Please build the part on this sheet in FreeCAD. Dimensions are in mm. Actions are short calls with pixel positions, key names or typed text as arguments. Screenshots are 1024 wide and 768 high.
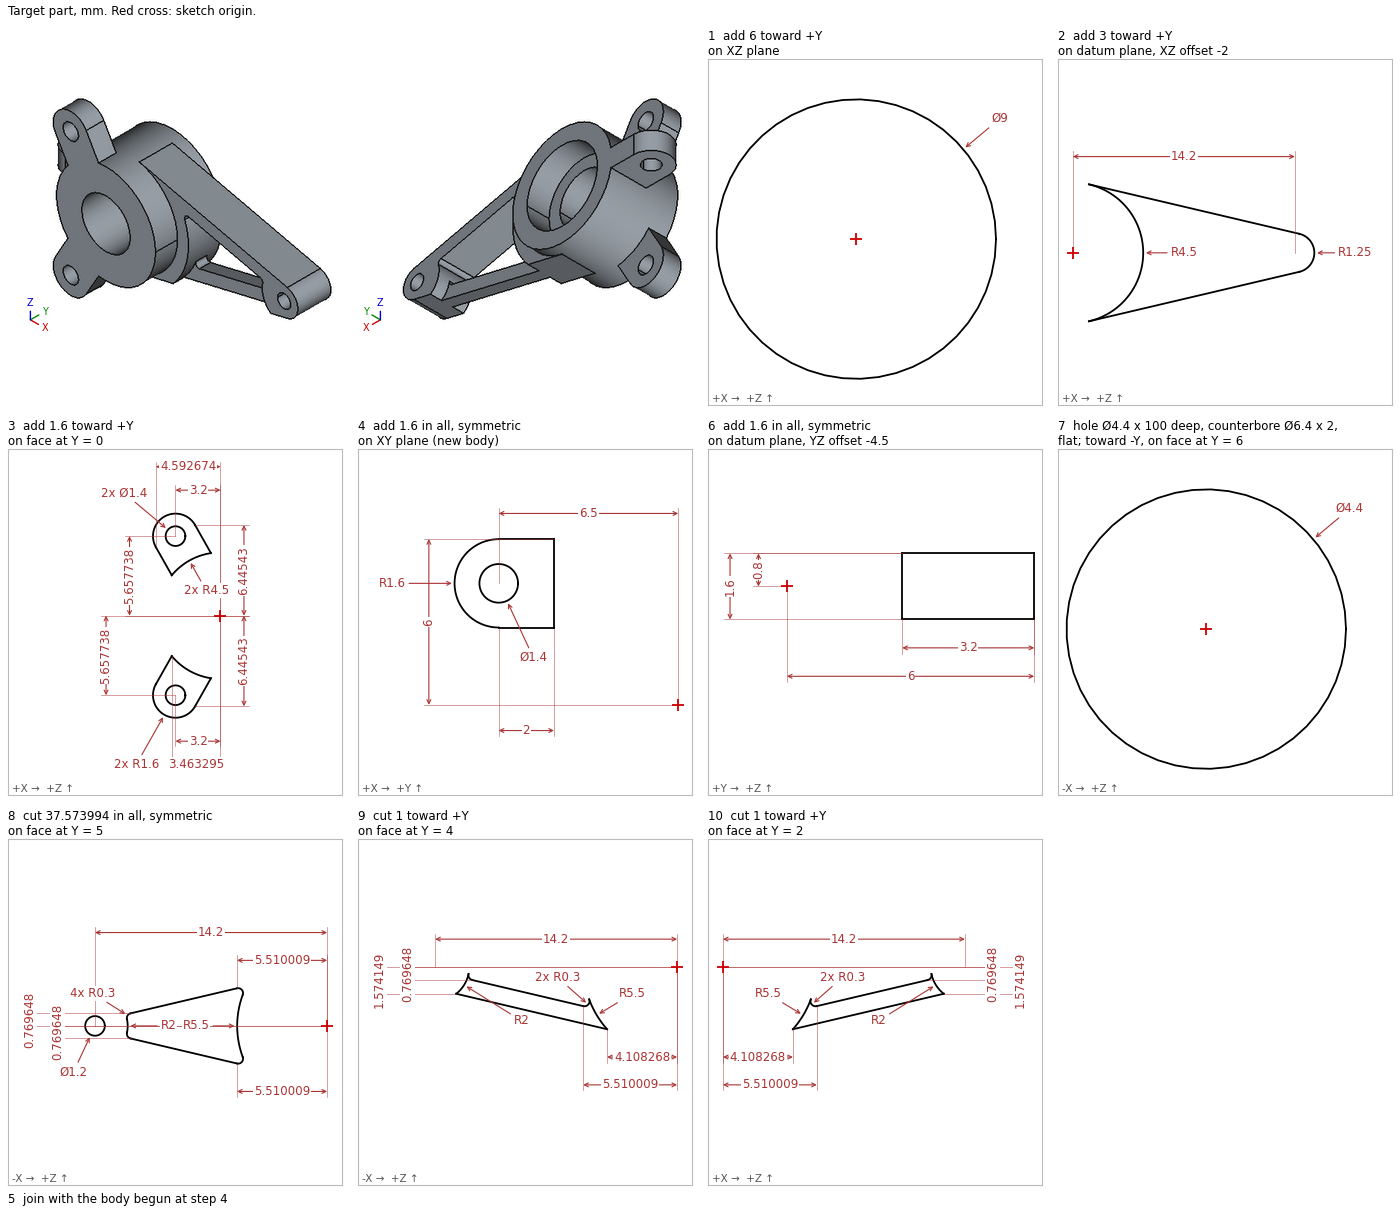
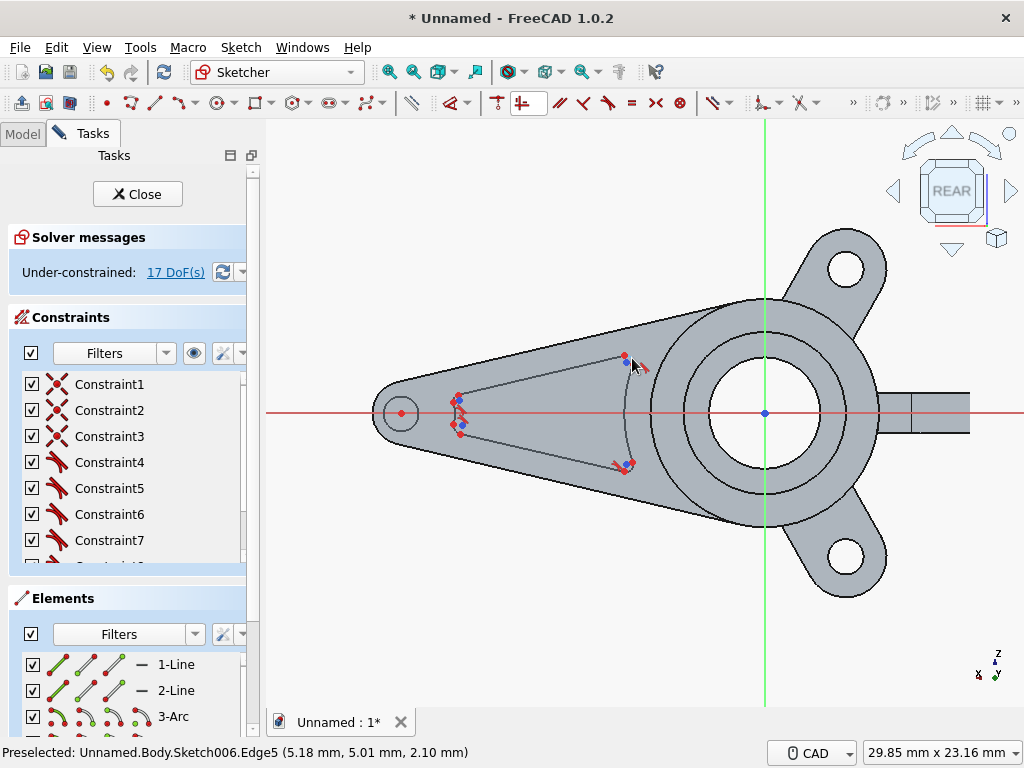
scroll(454, 398, up, 6)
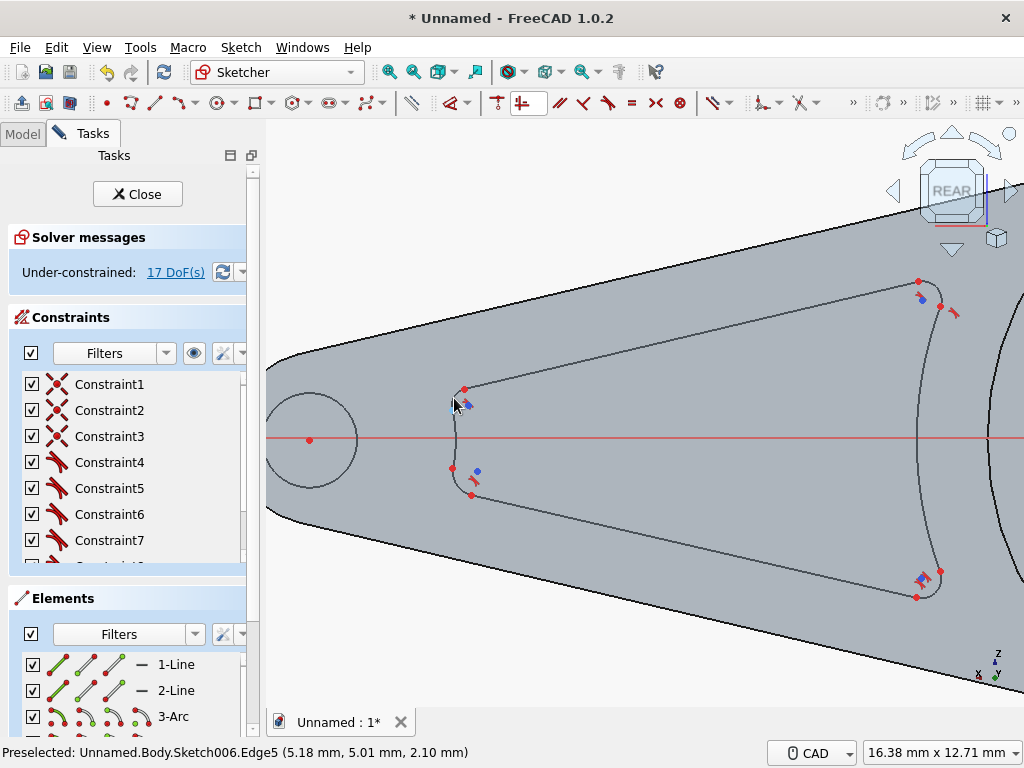
click(454, 397)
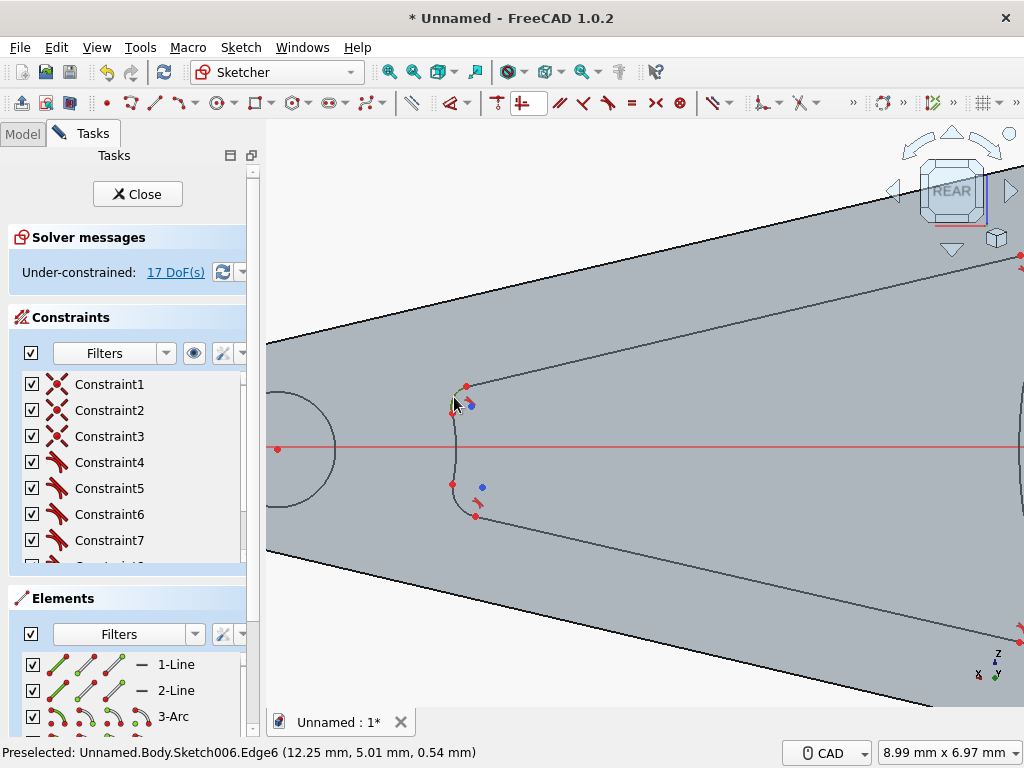
click(456, 463)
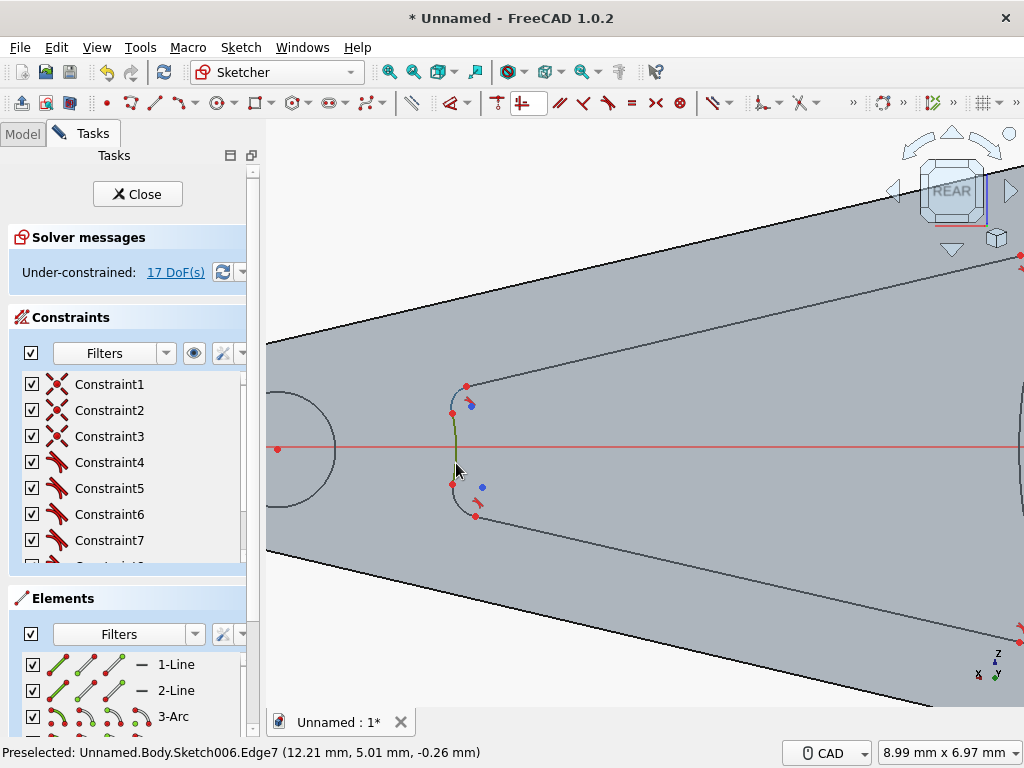
key(t)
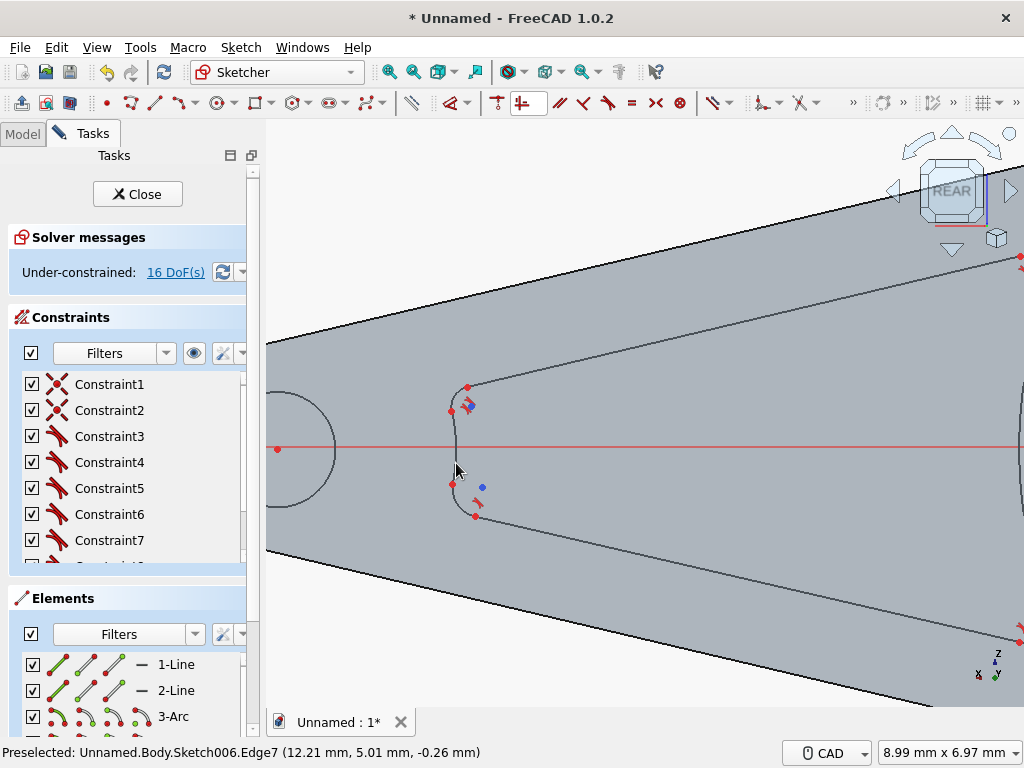
click(456, 462)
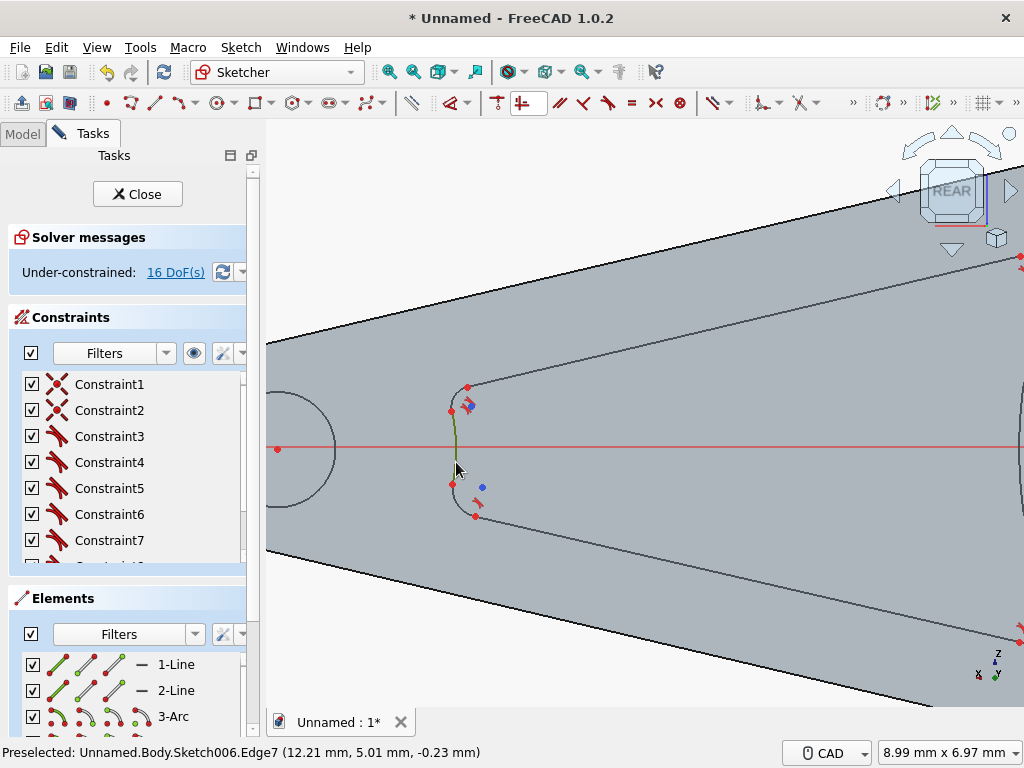
click(454, 497)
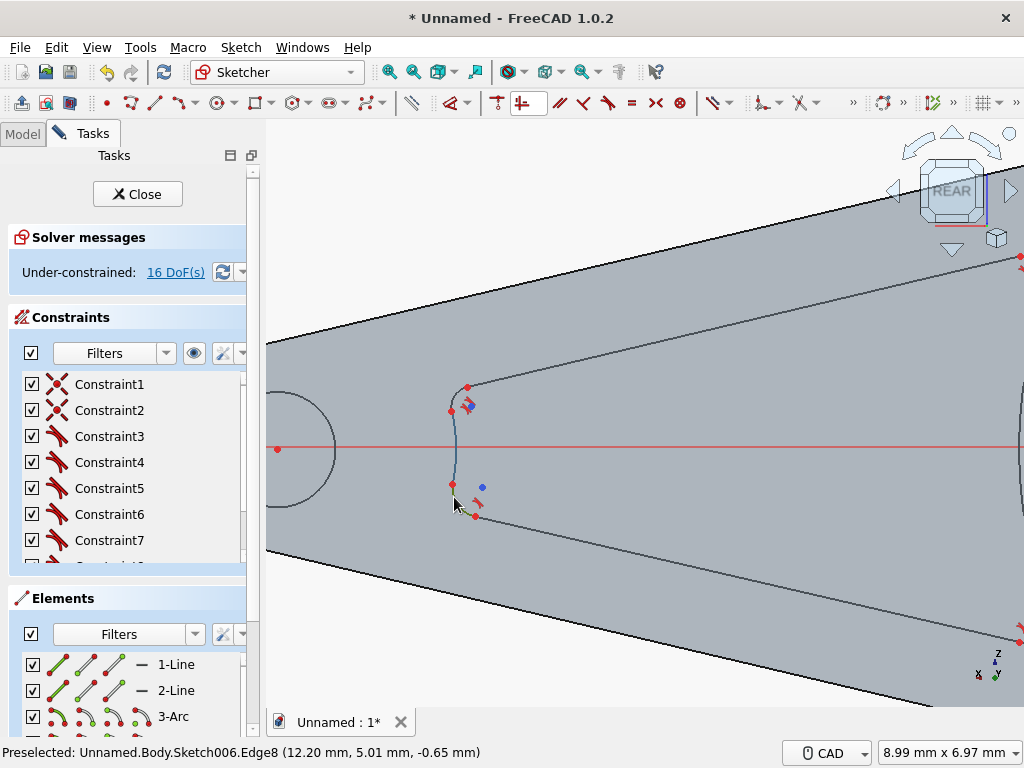
click(608, 104)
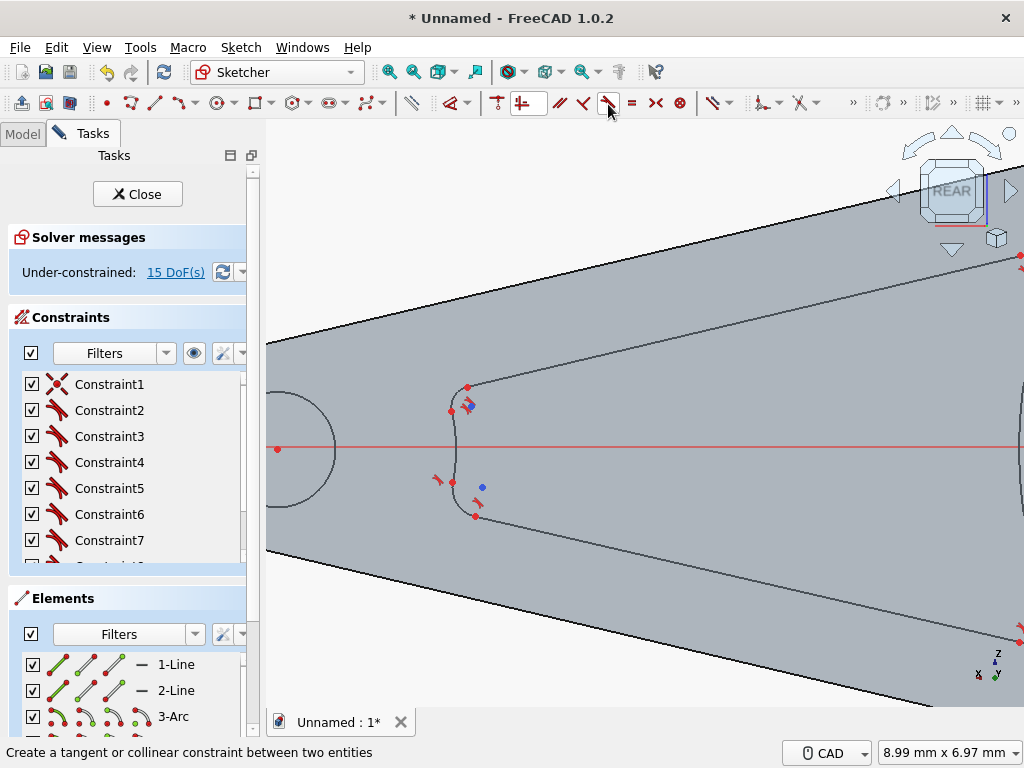
scroll(454, 398, down, 6)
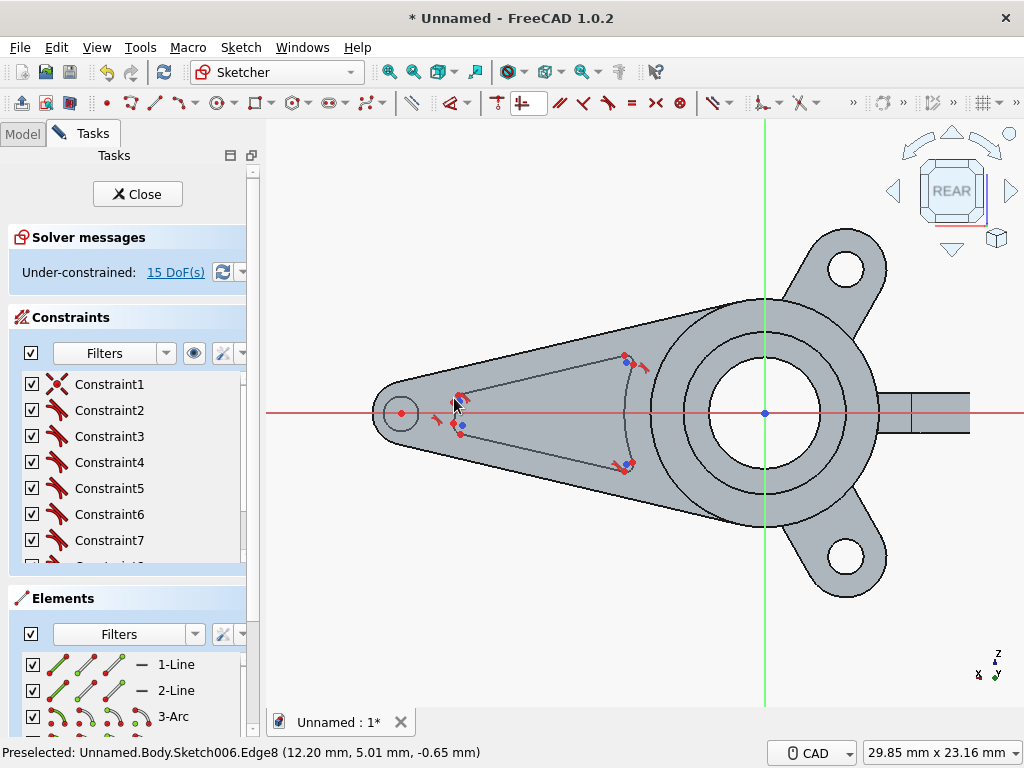
scroll(765, 413, up, 10)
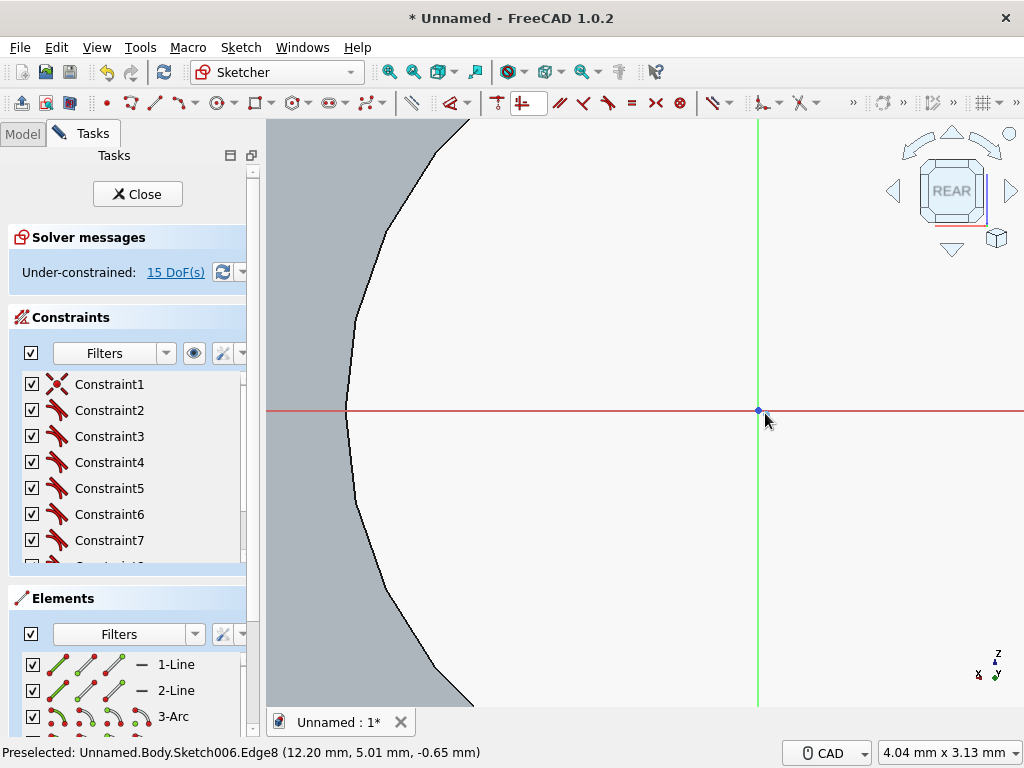
drag(748, 401, 777, 425)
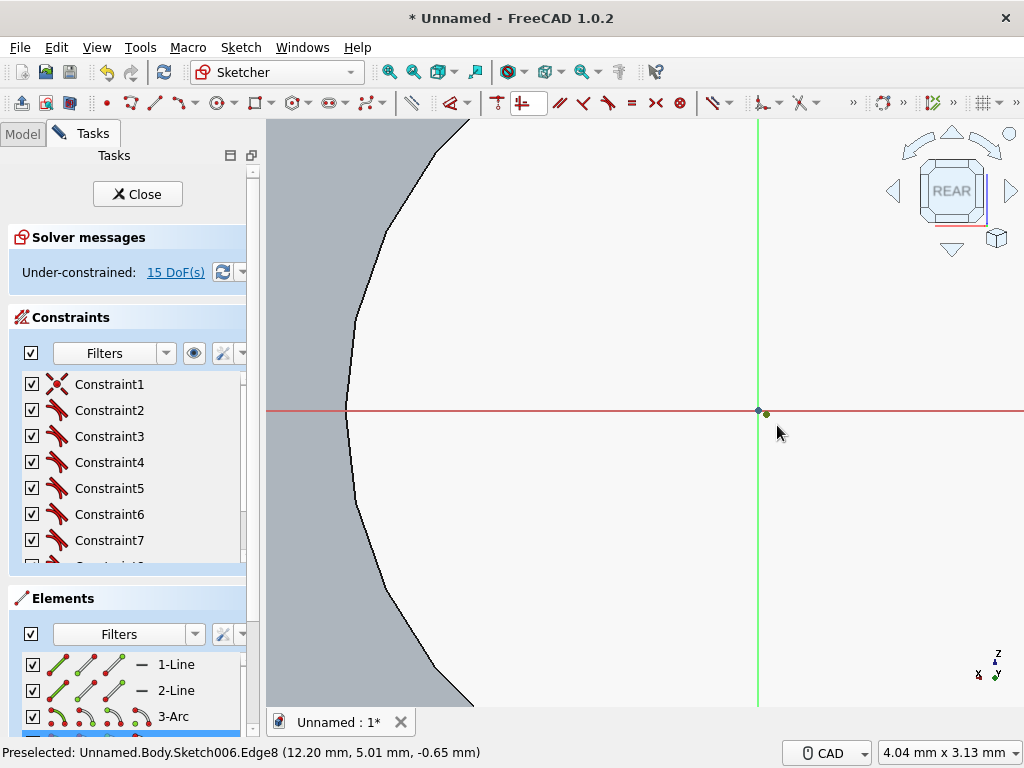
key(c)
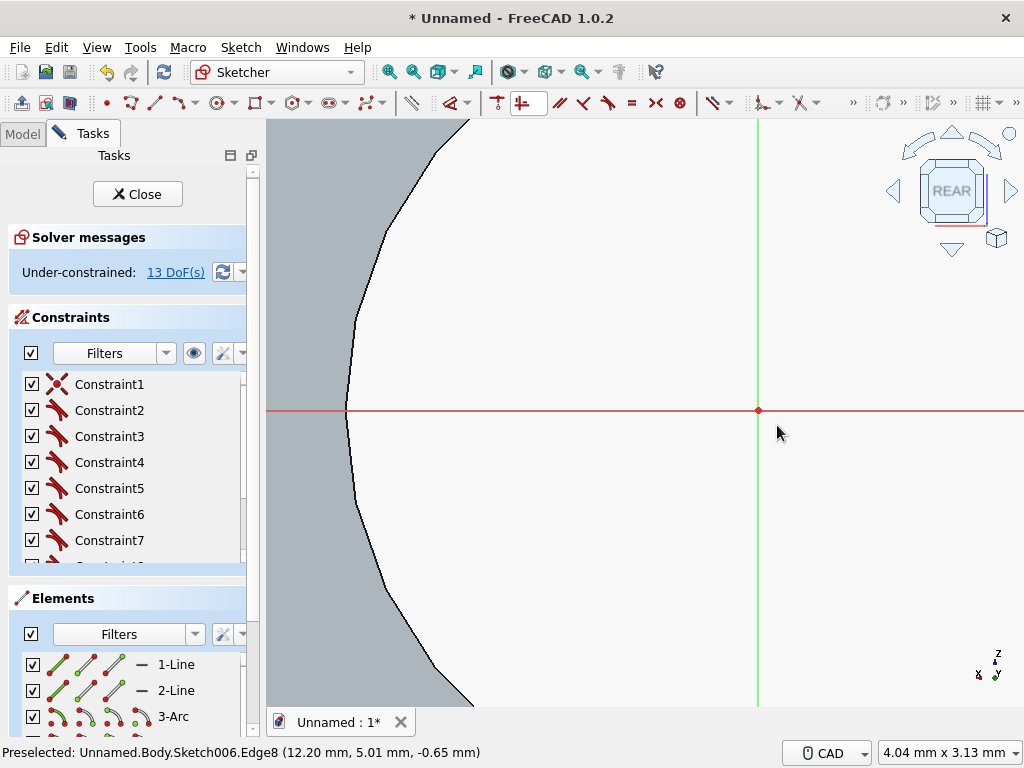
scroll(765, 413, down, 10)